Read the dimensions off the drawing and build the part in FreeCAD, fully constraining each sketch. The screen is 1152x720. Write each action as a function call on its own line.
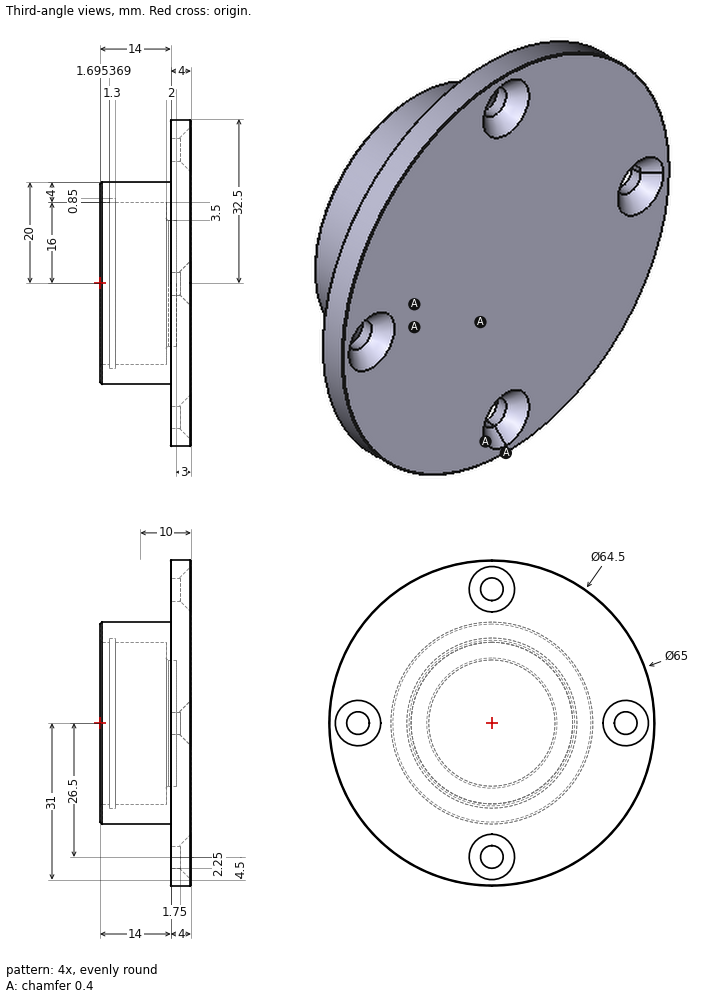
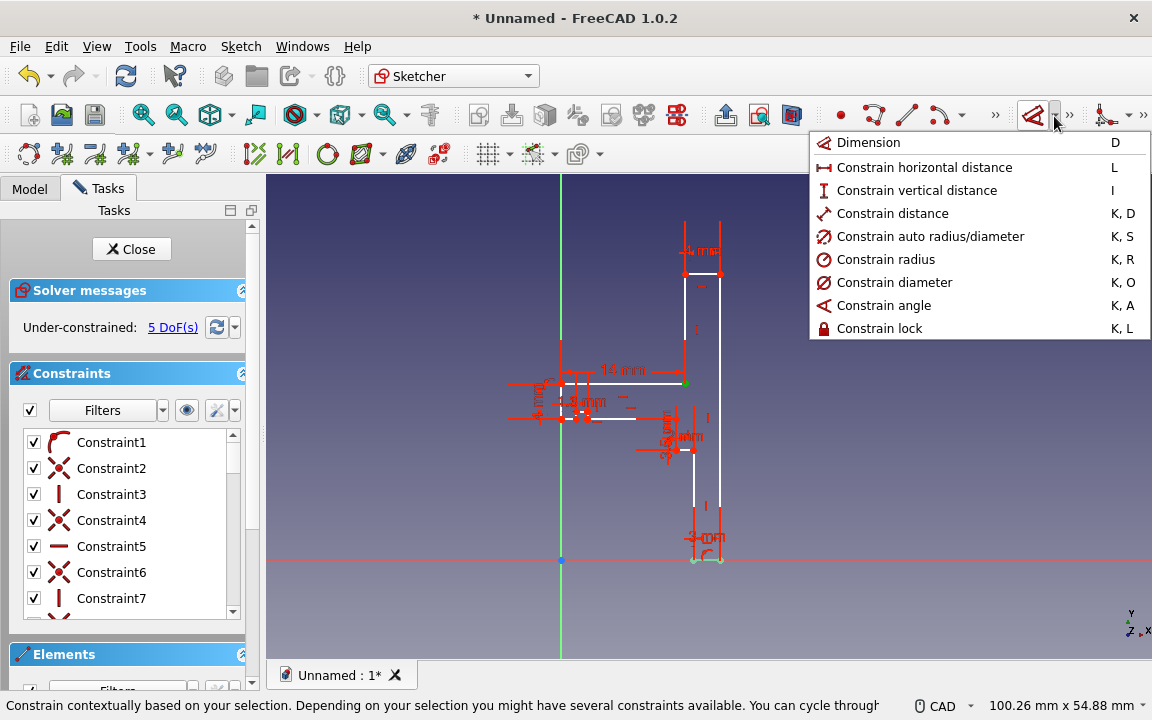
click(980, 190)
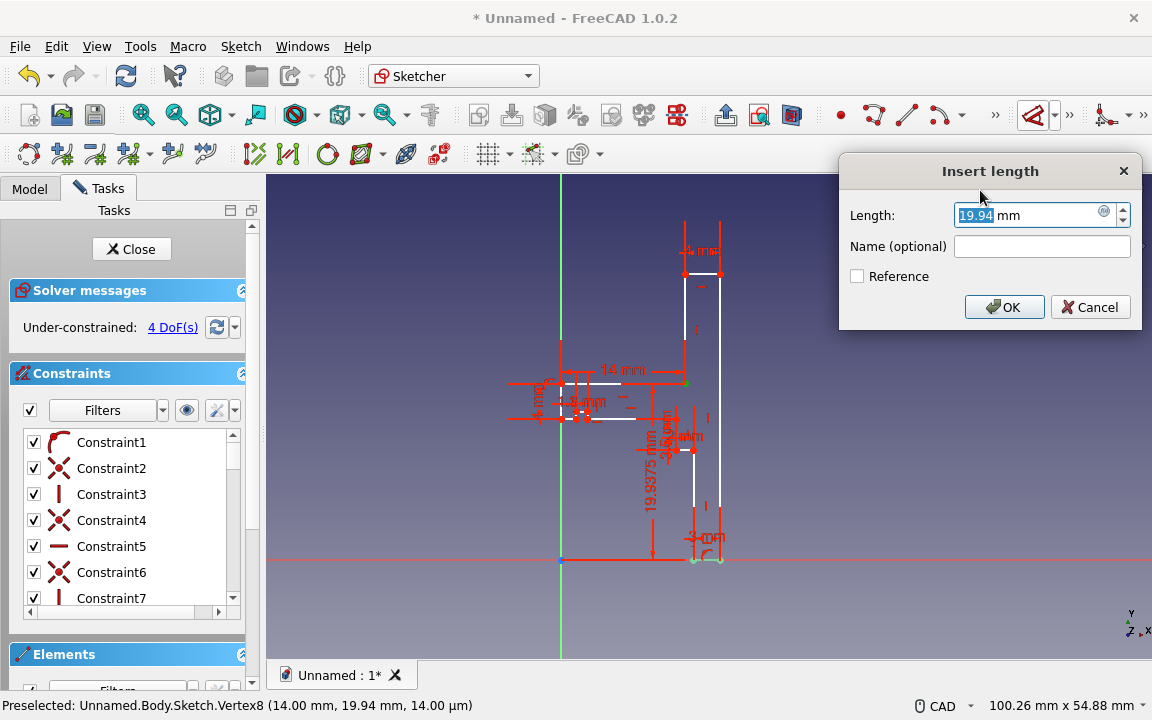
text(20)
key(Return)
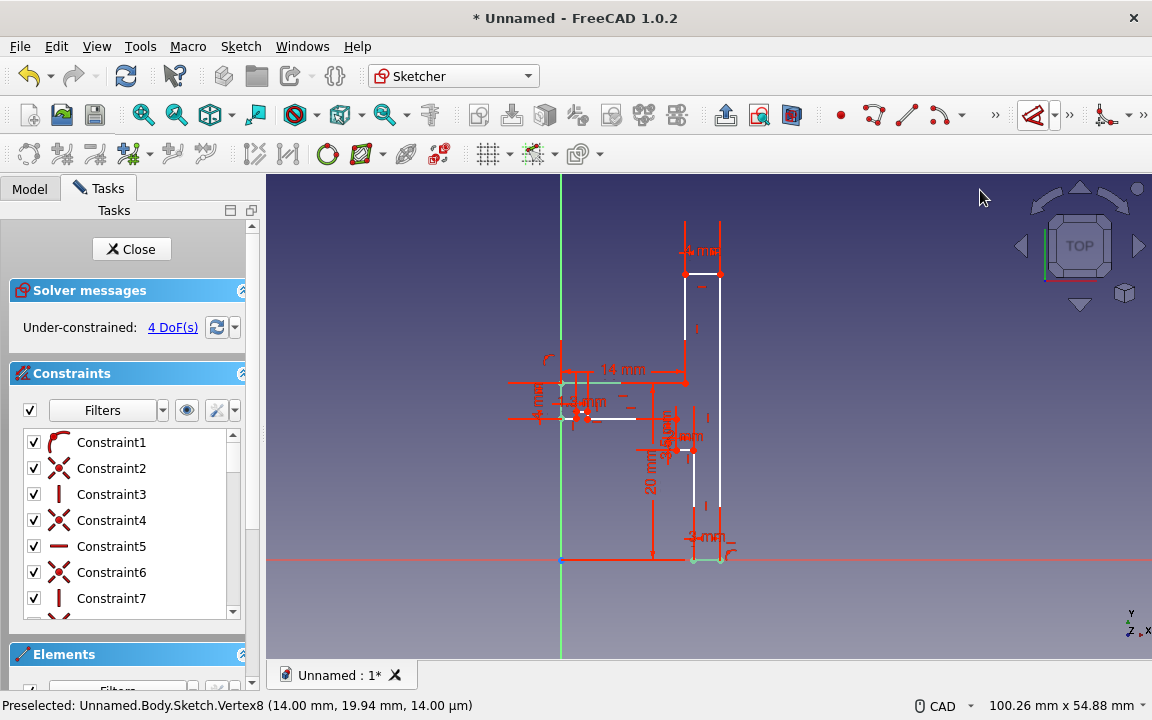
scroll(588, 419, up, 3)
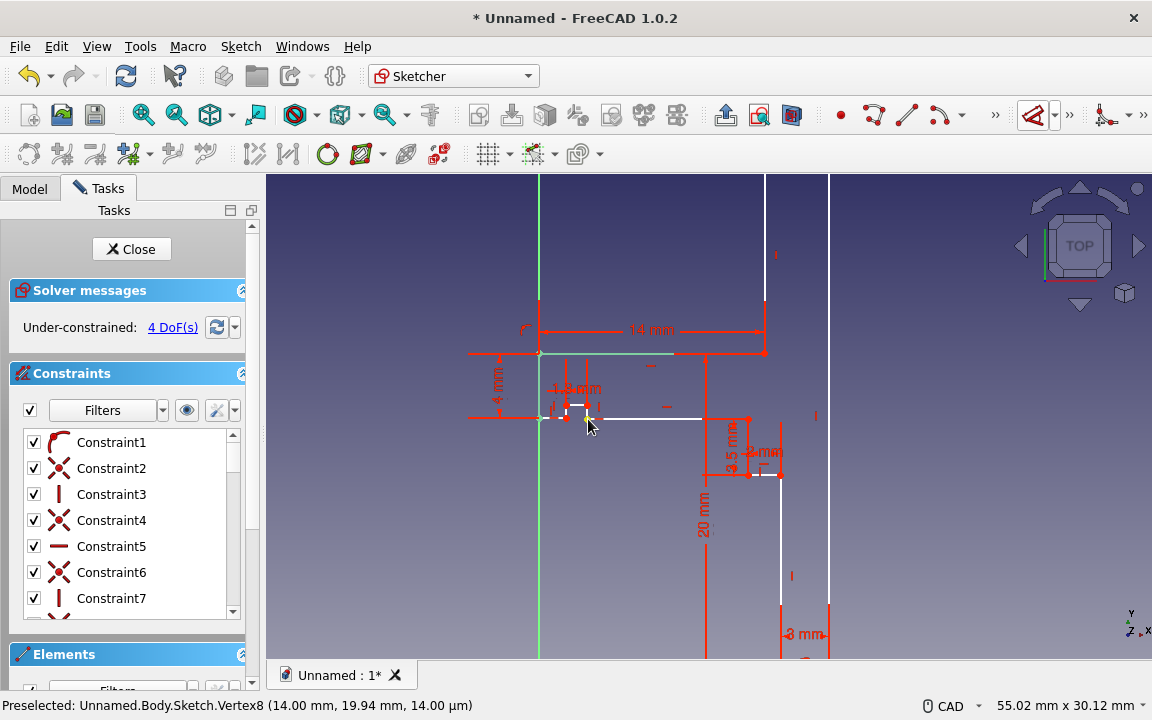
click(587, 419)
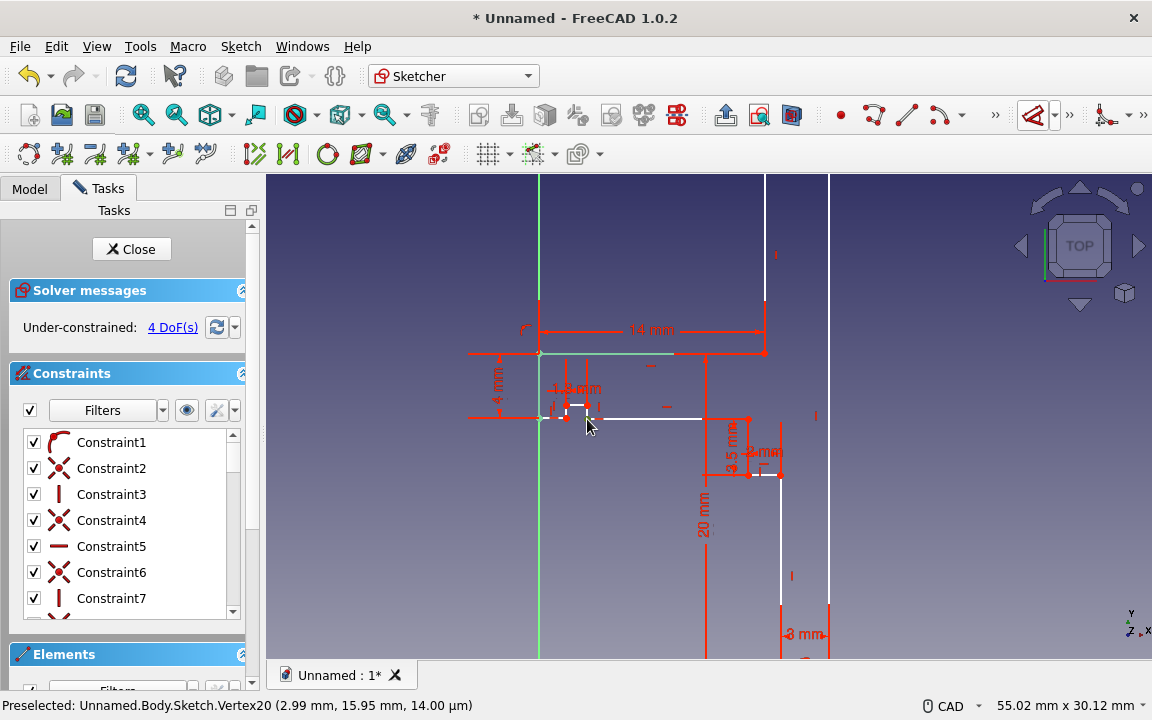
click(1054, 116)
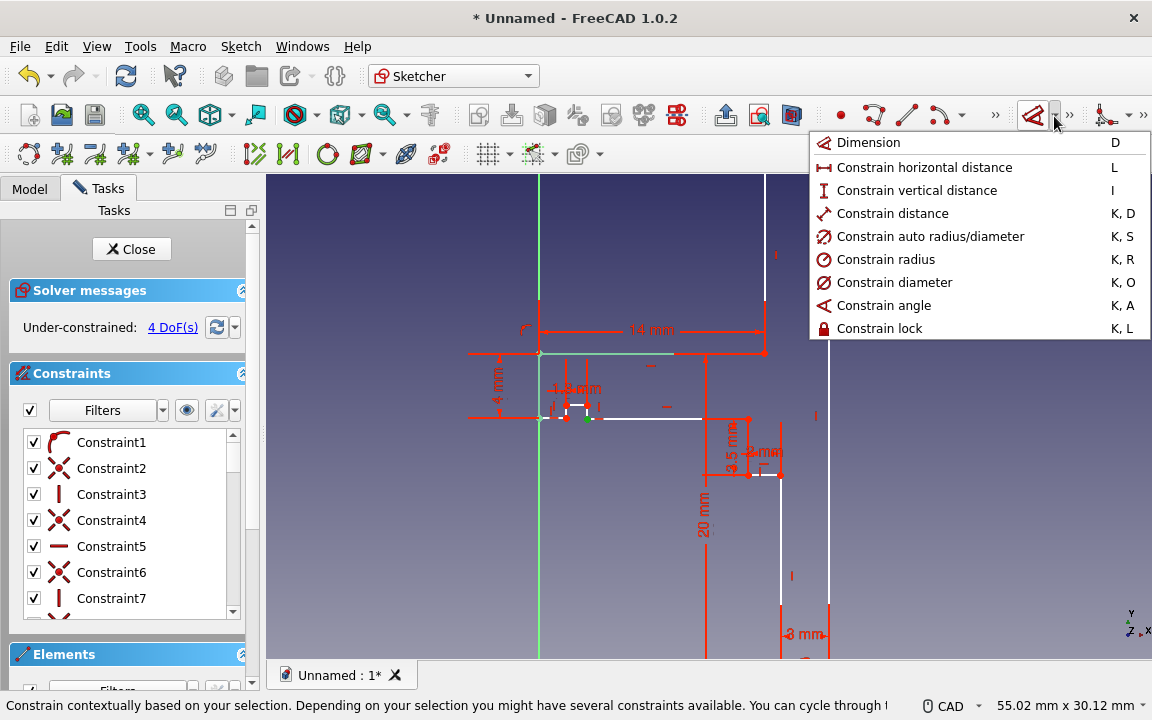
click(980, 190)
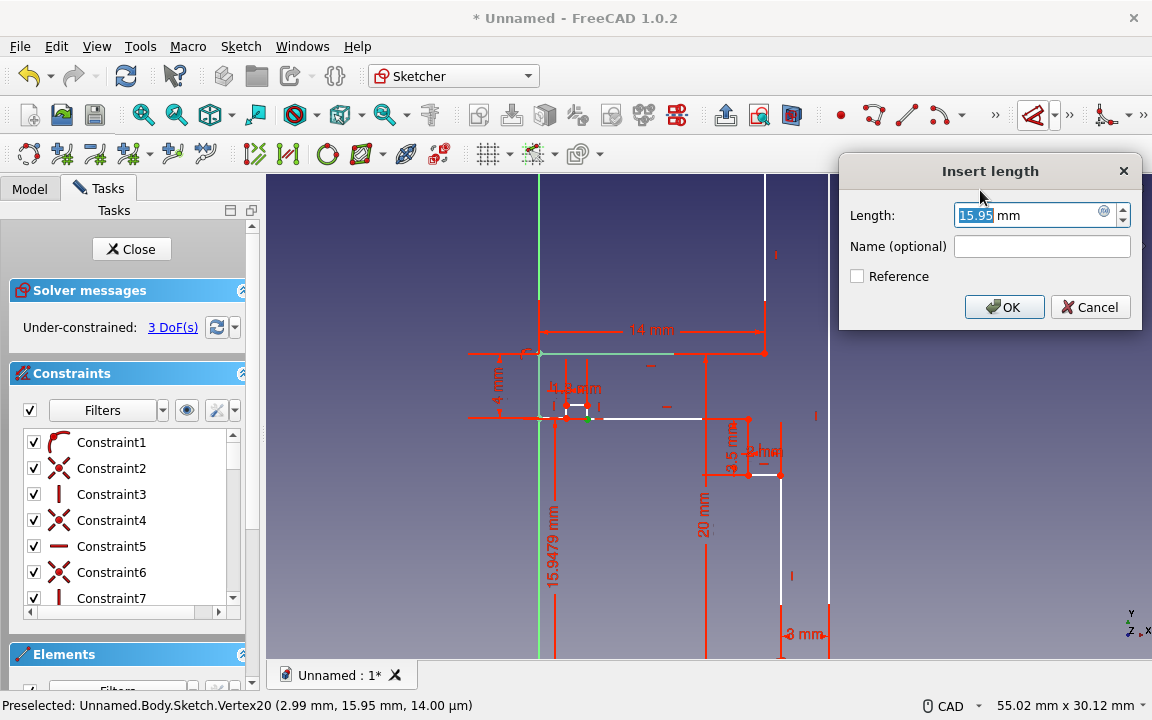
text(16)
key(Return)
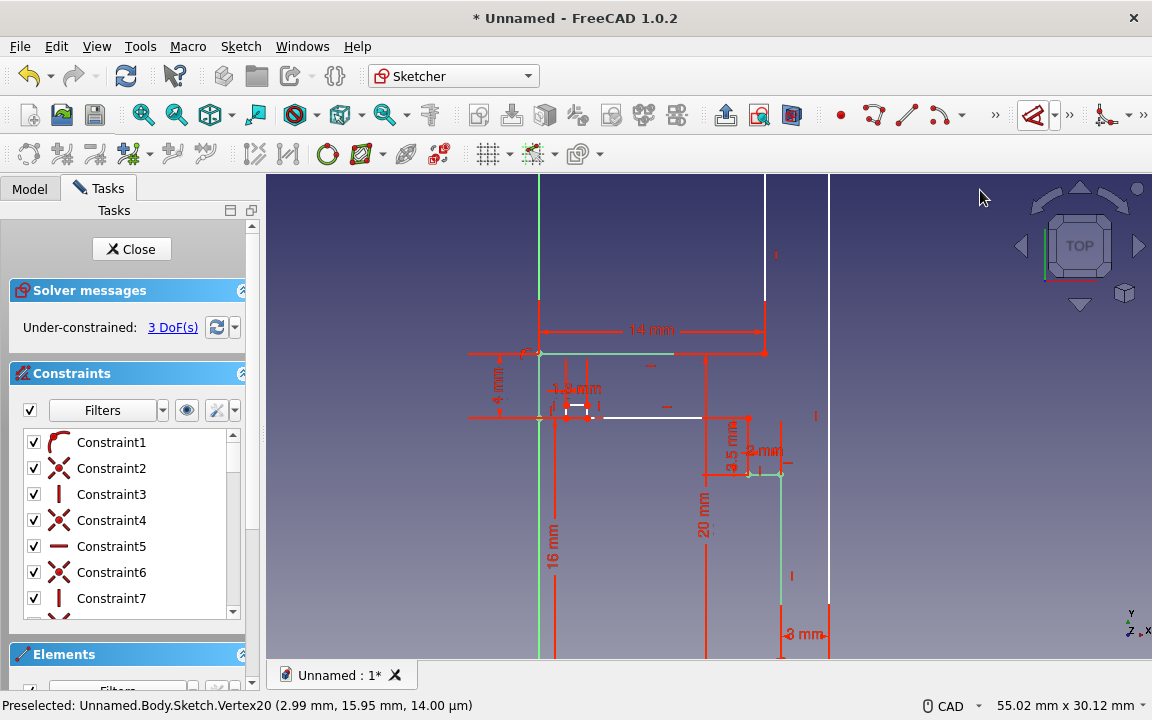
click(829, 520)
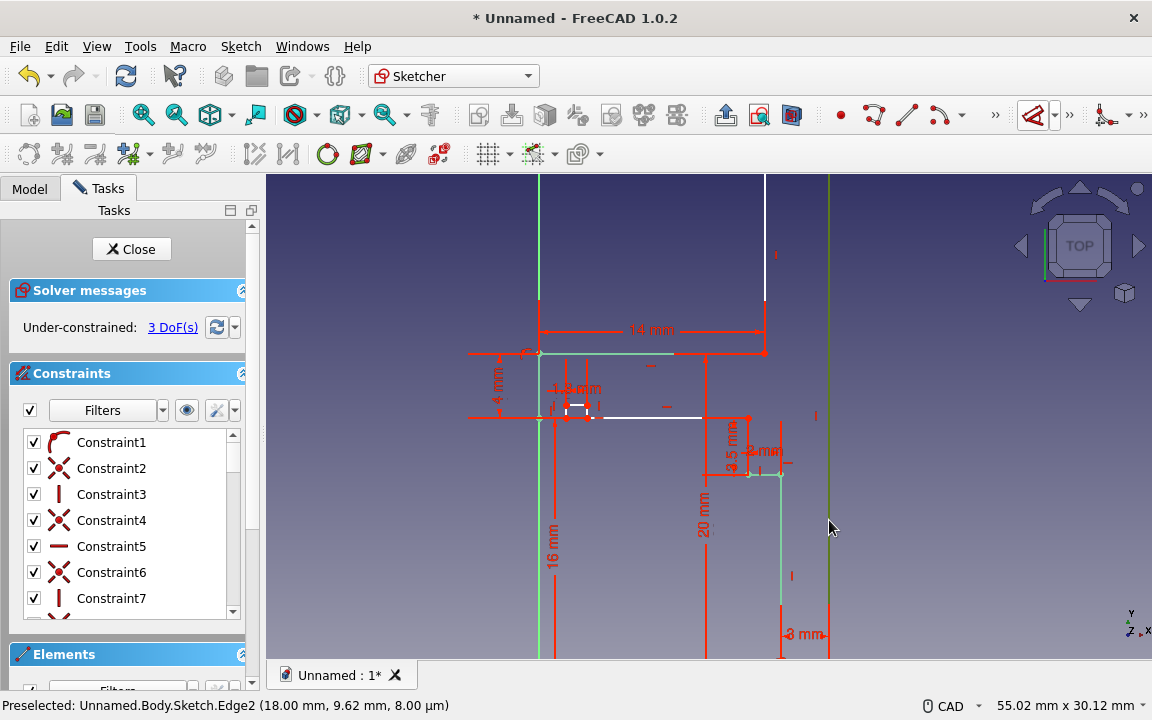
key(i)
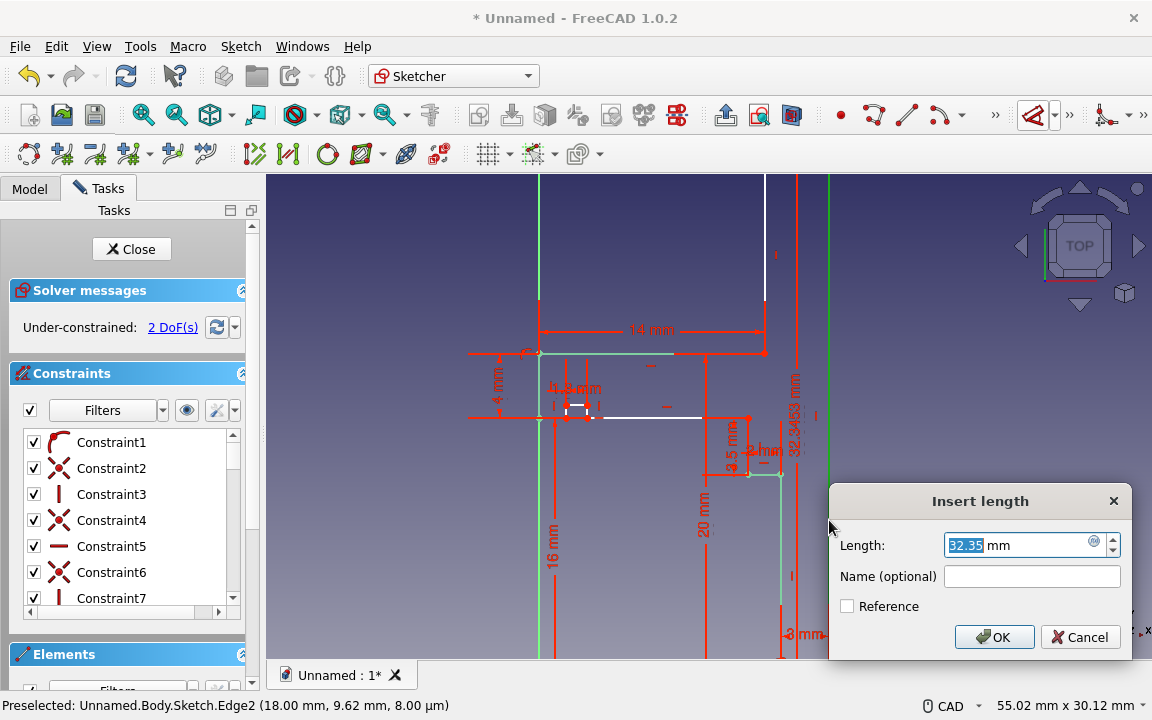
text(32.5)
key(Return)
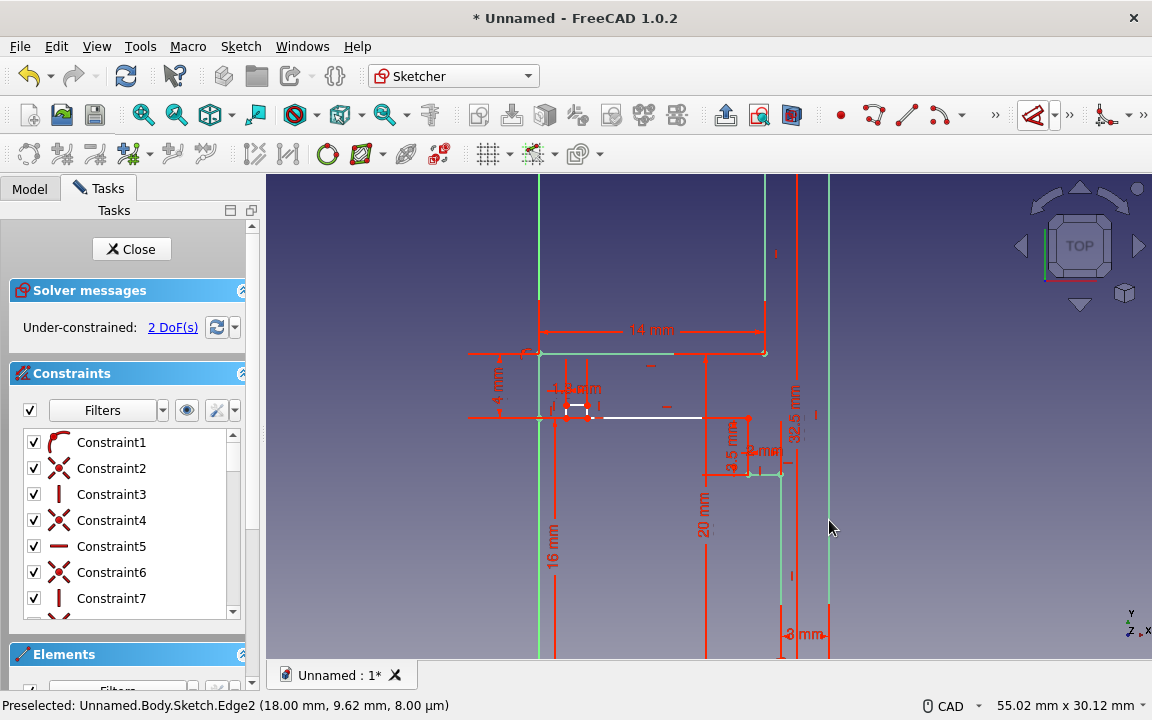
scroll(566, 412, up, 6)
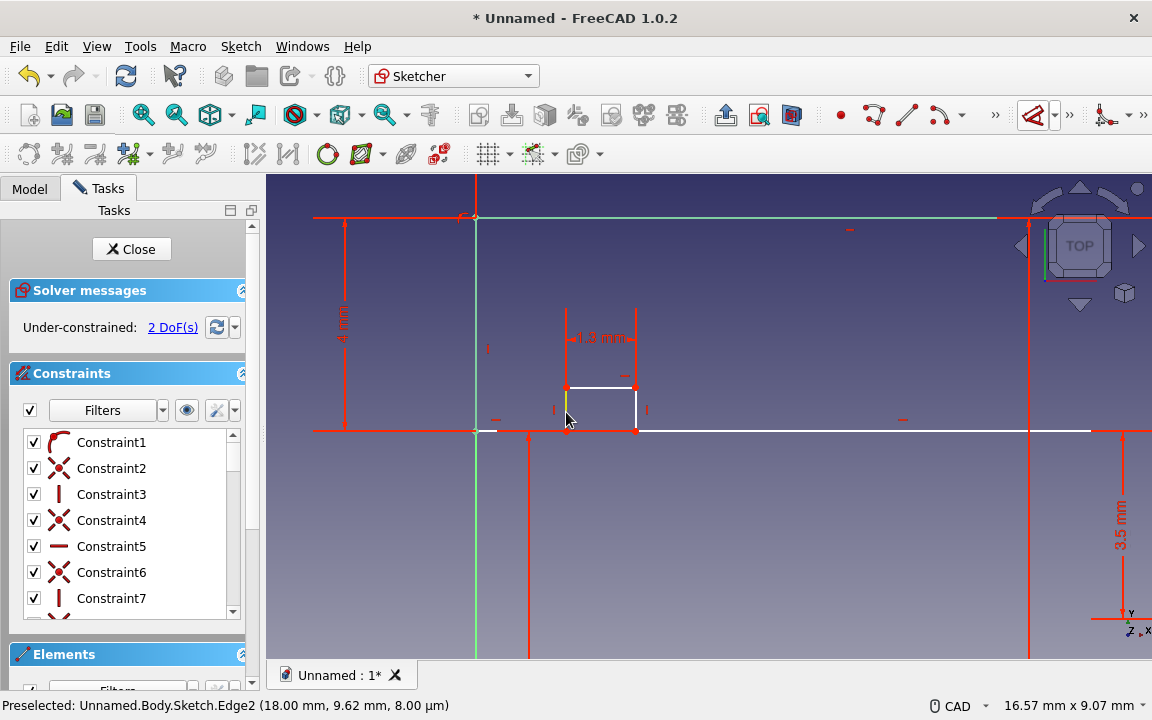
click(566, 410)